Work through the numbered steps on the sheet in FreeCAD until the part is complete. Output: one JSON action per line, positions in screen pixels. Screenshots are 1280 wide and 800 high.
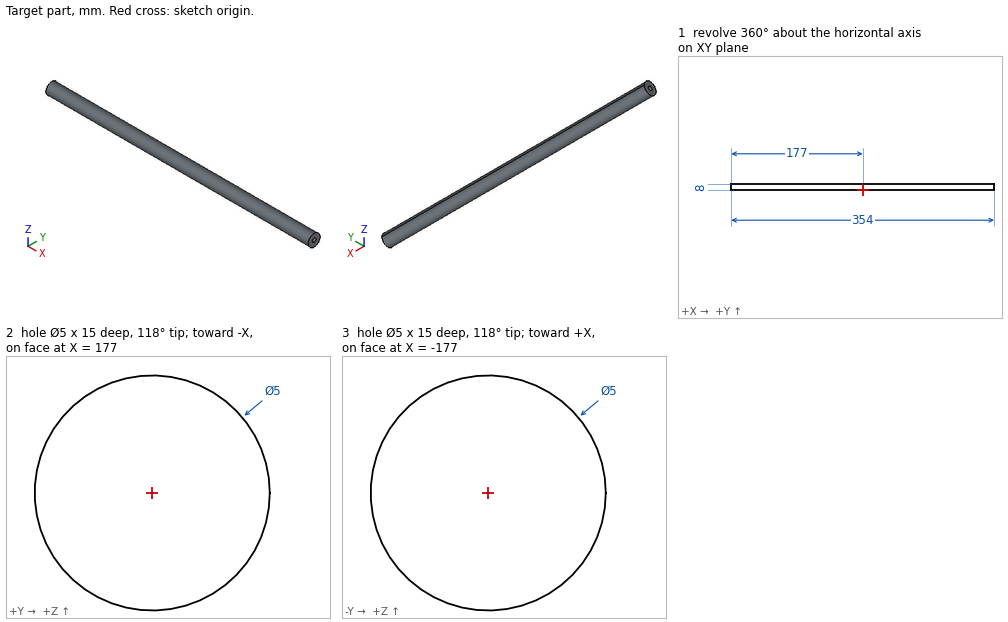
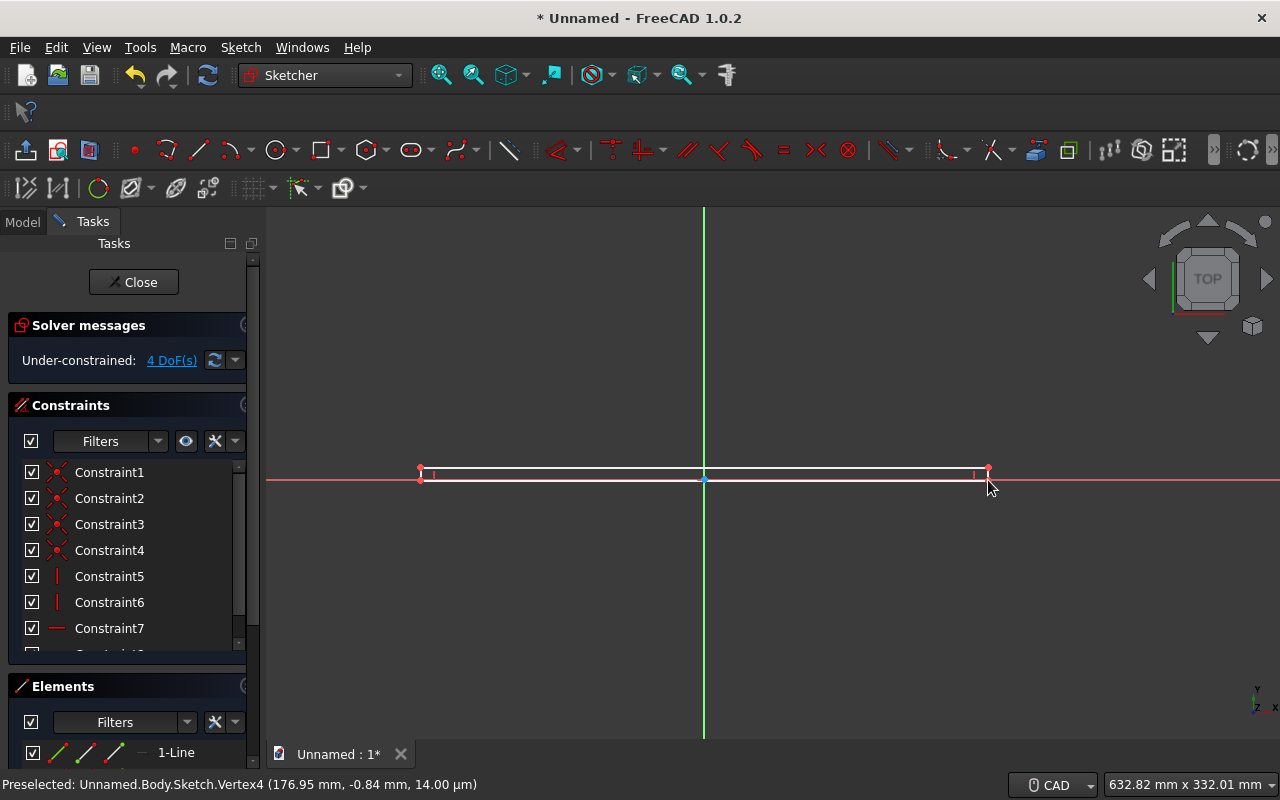
{"action": "left_click", "coordinate": [421, 481]}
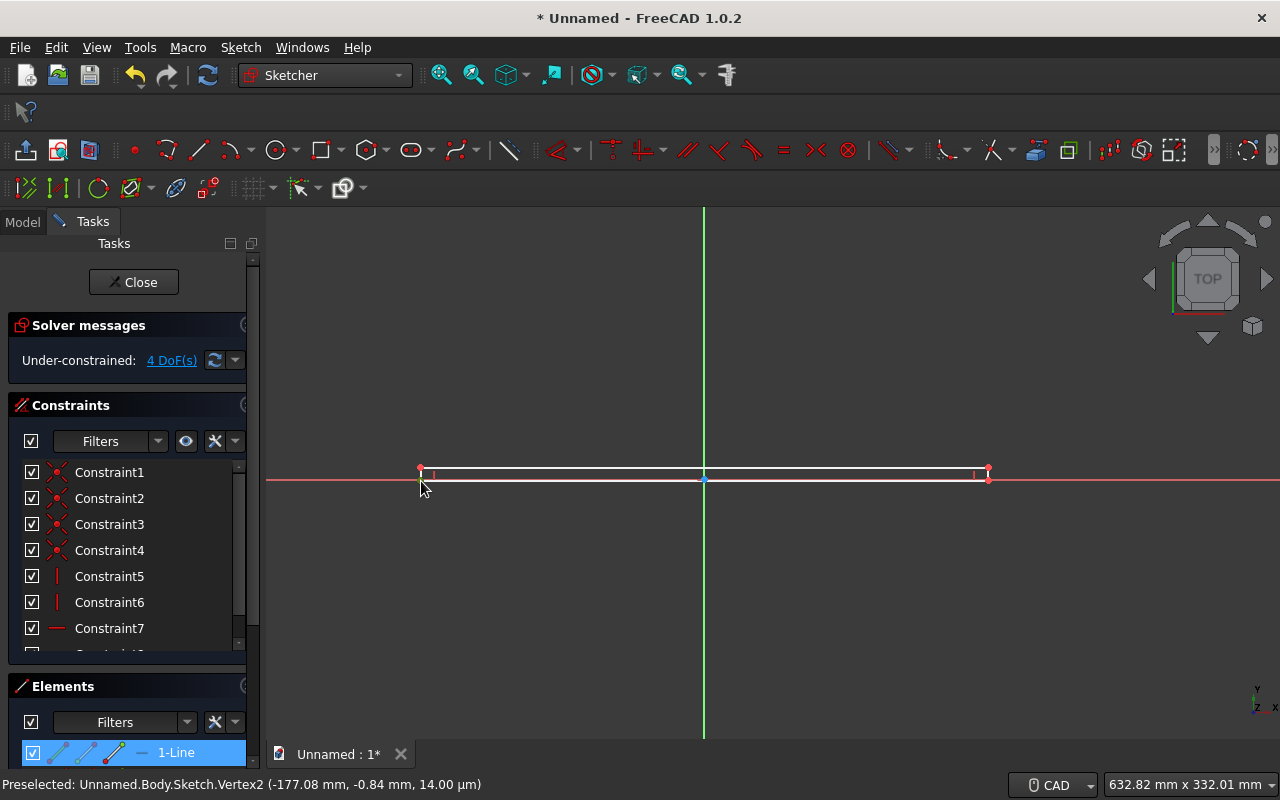
{"action": "left_click", "coordinate": [353, 480]}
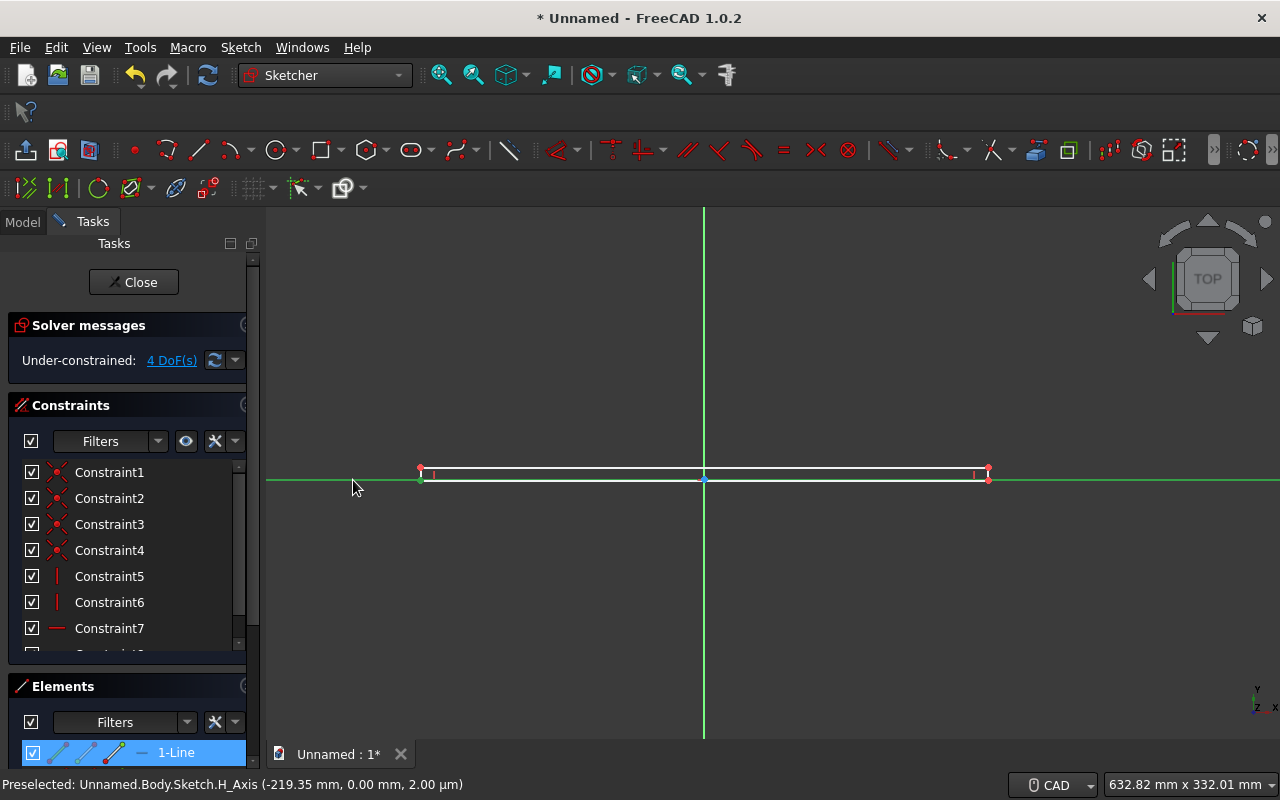
{"action": "left_click", "coordinate": [612, 150]}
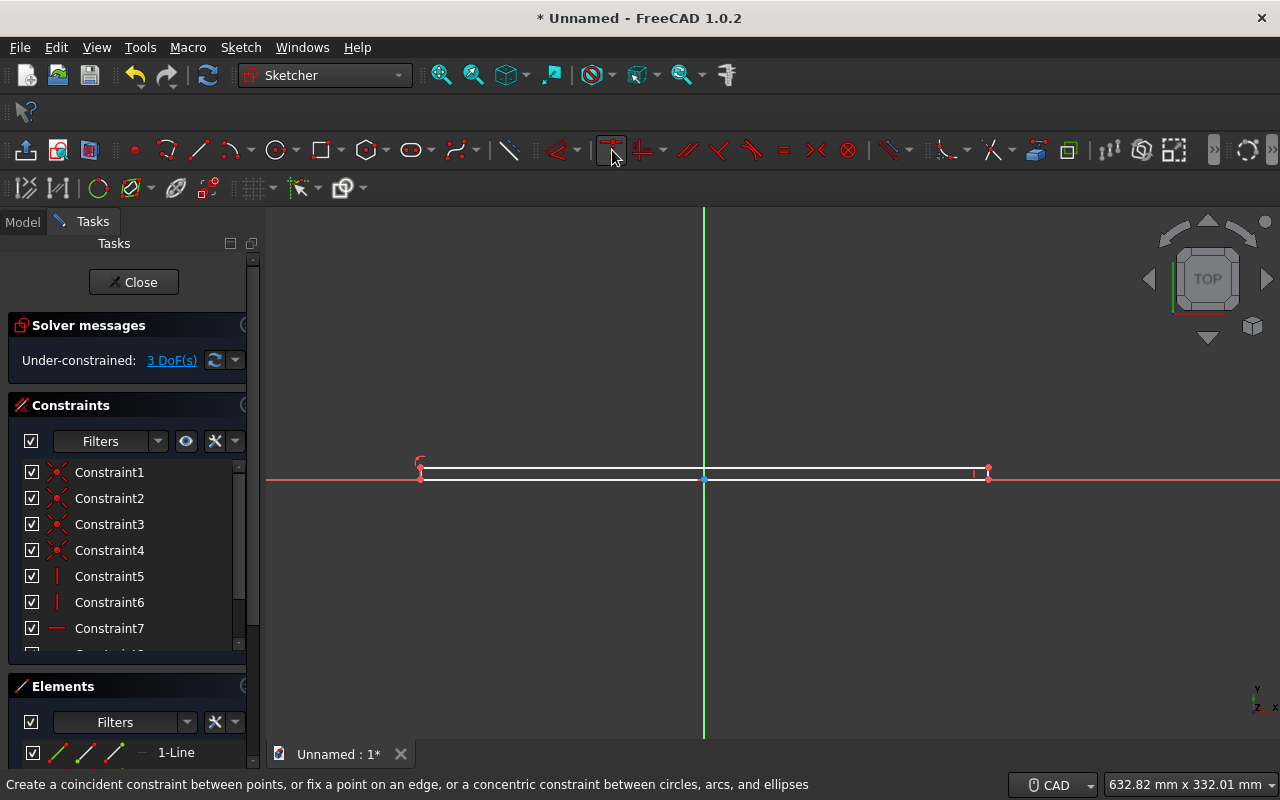
{"action": "key", "text": "d"}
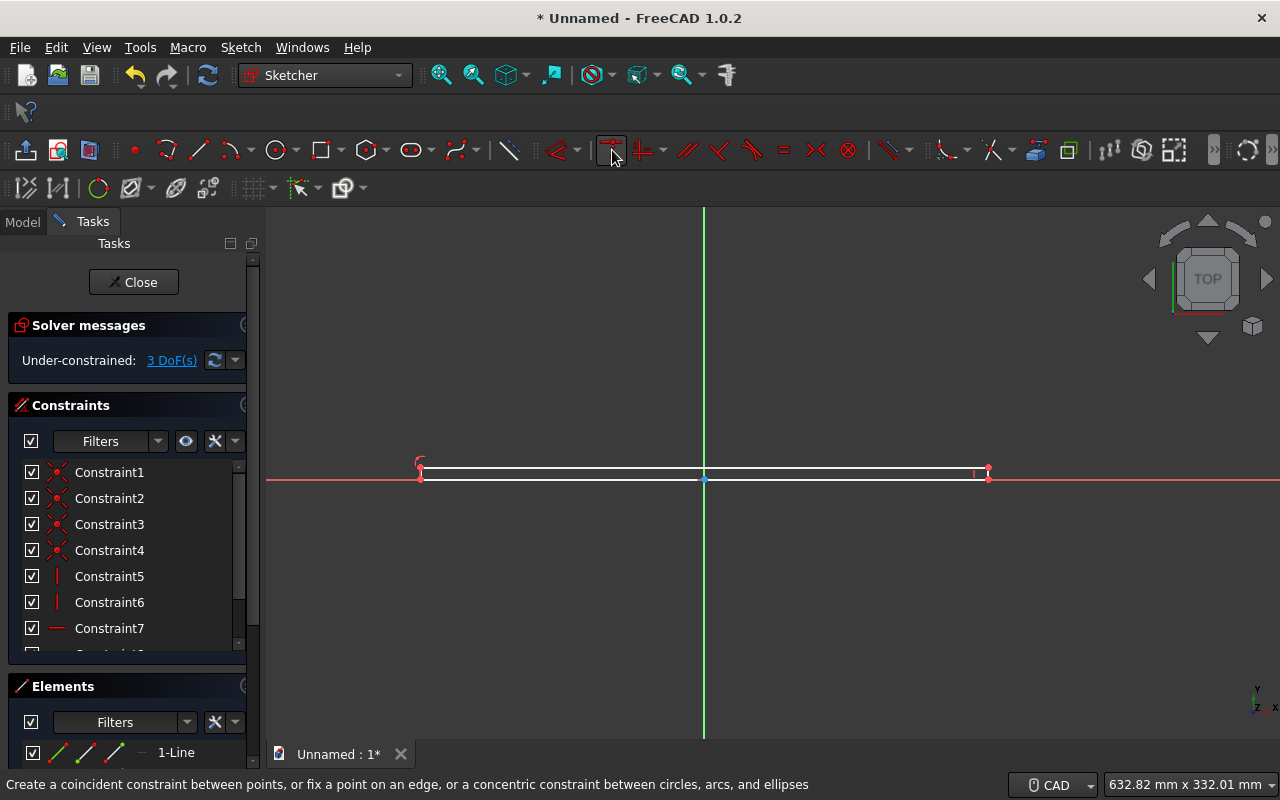
{"action": "scroll", "coordinate": [421, 474], "scroll_direction": "up", "scroll_amount": 6}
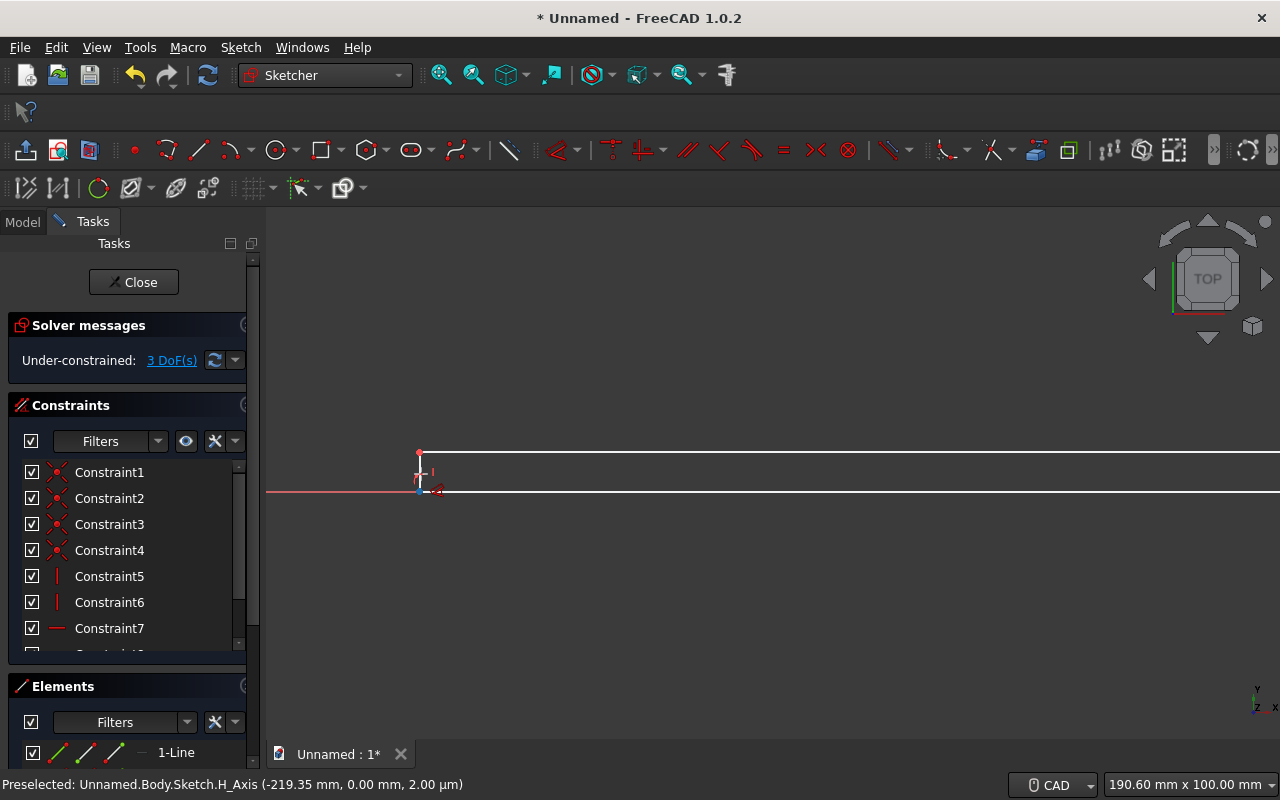
{"action": "left_click", "coordinate": [420, 472]}
{"action": "left_click", "coordinate": [386, 472]}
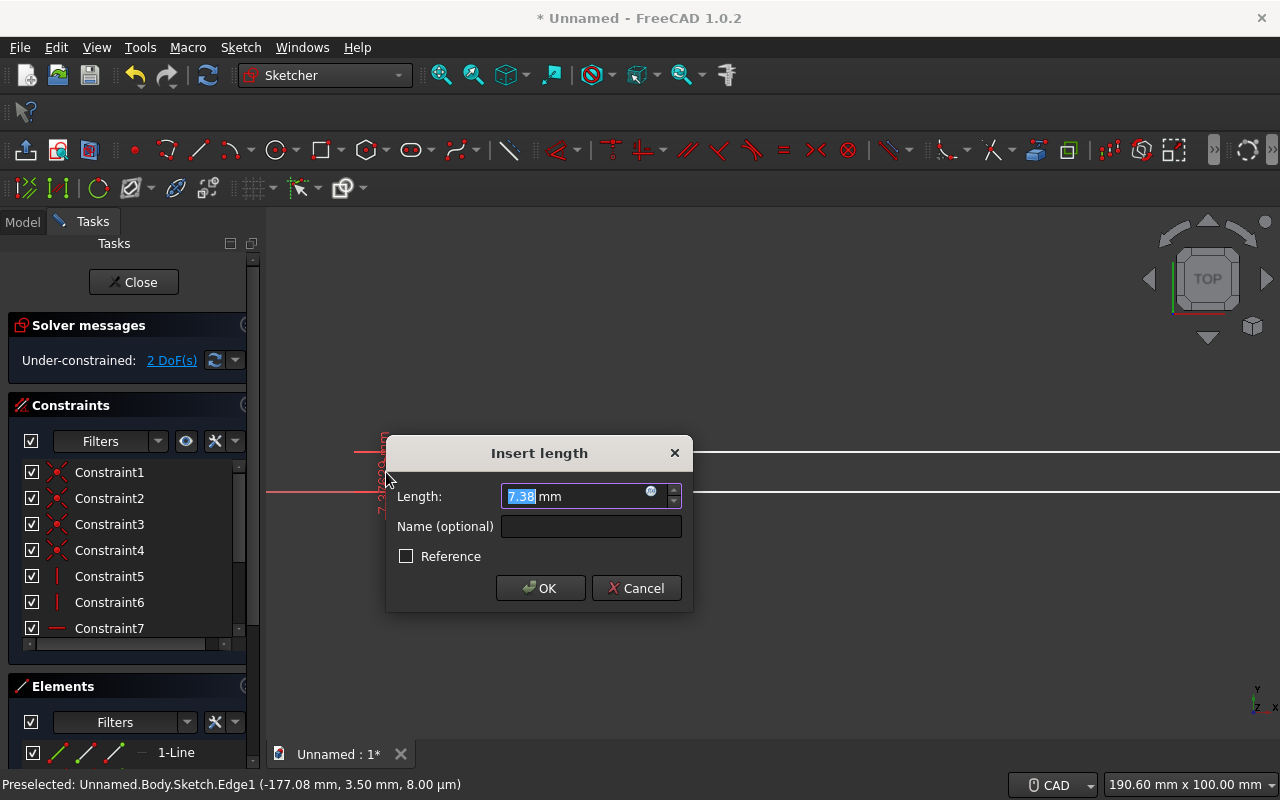
{"action": "type", "text": "8"}
{"action": "key", "text": "Return"}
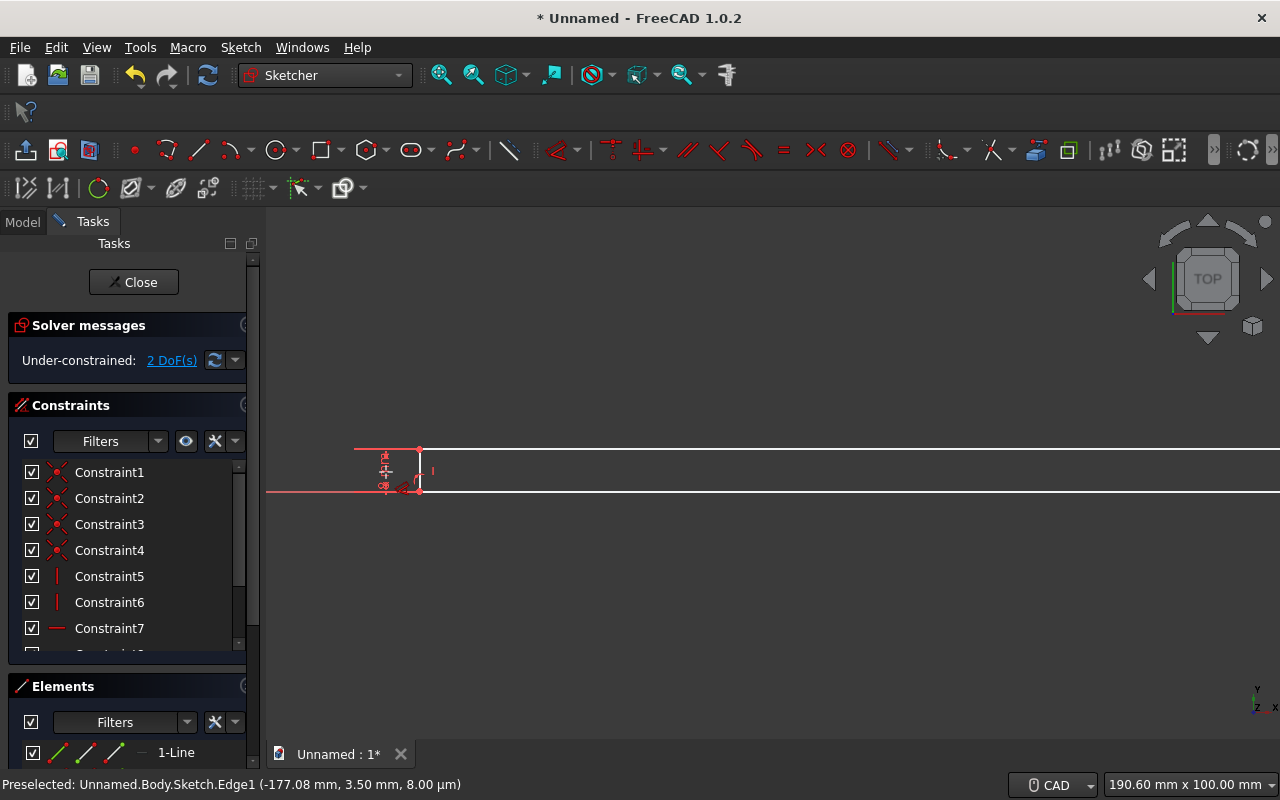
{"action": "left_click", "coordinate": [985, 492]}
{"action": "left_click", "coordinate": [767, 526]}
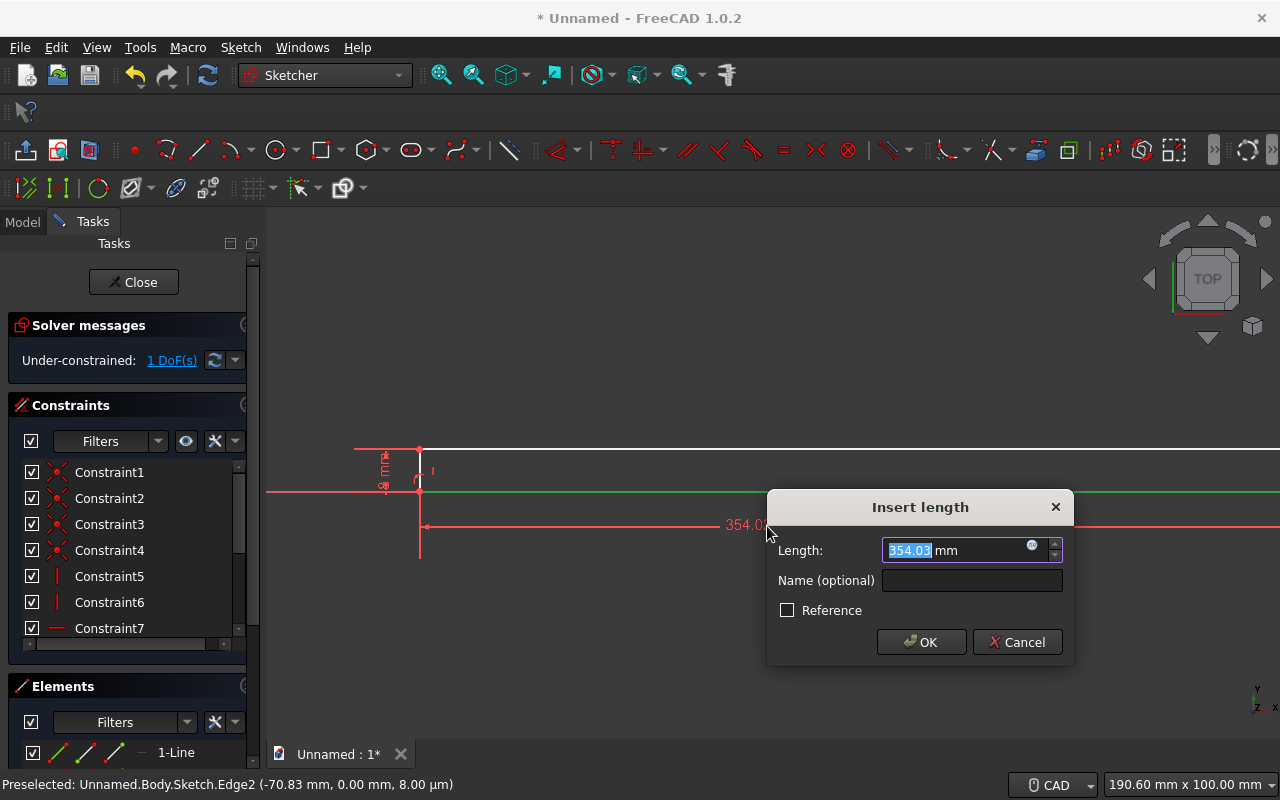
{"action": "type", "text": "354"}
{"action": "key", "text": "Return"}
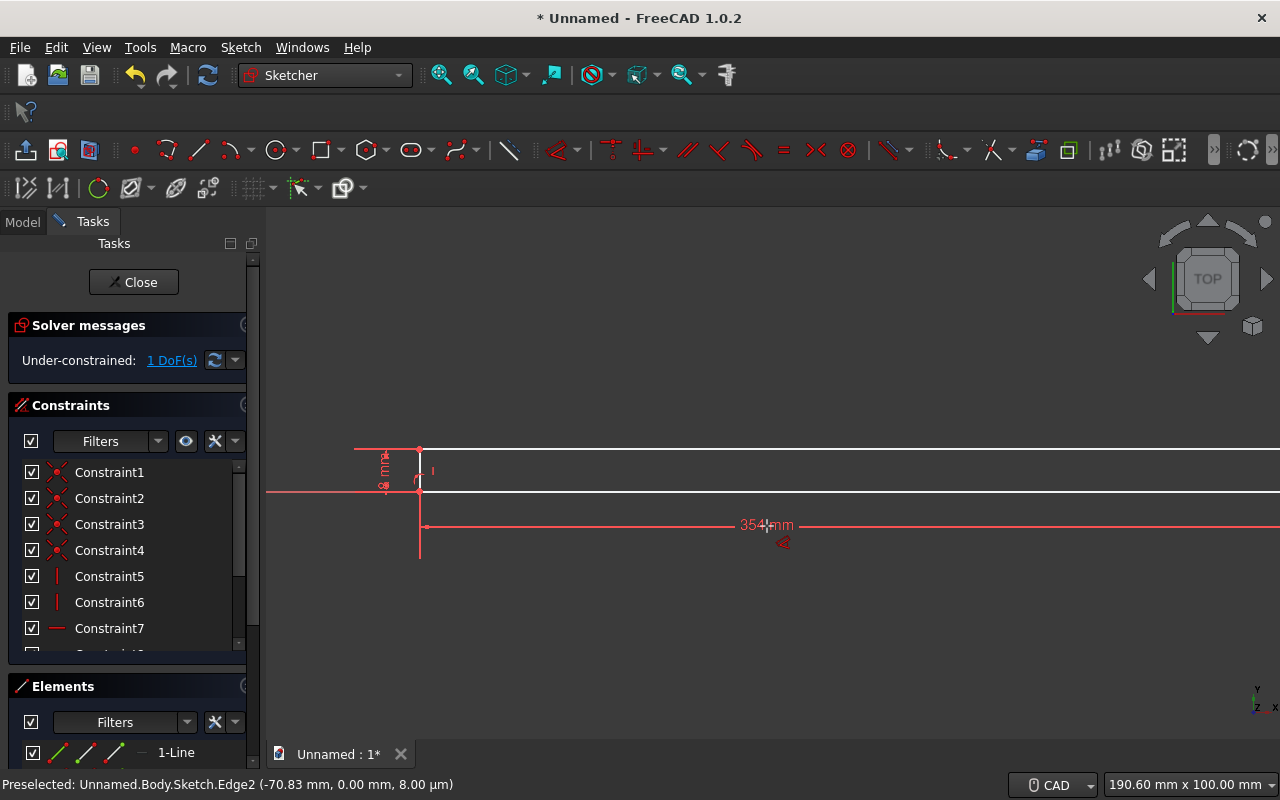
{"action": "left_click", "coordinate": [420, 449]}
{"action": "left_click", "coordinate": [608, 526]}